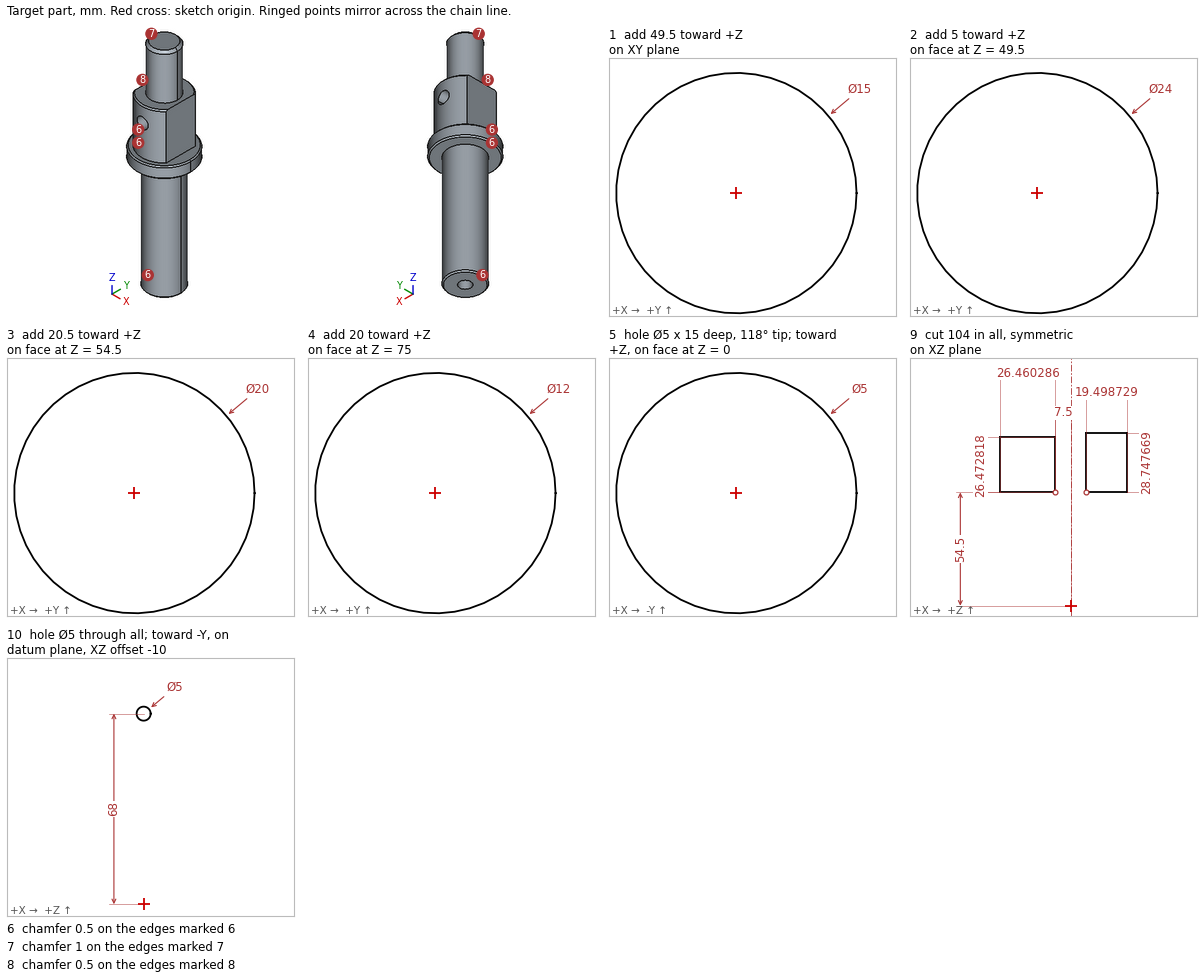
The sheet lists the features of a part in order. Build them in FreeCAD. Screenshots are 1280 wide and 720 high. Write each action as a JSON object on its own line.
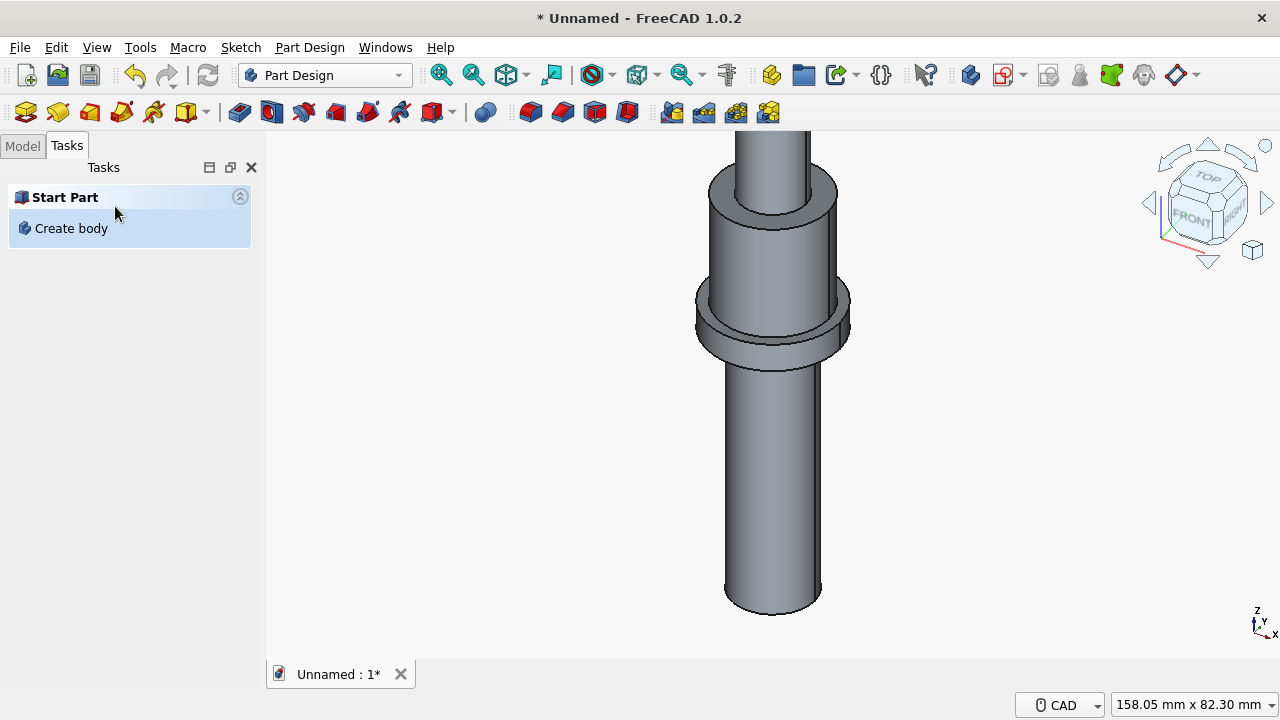
{"action": "left_click", "coordinate": [442, 76]}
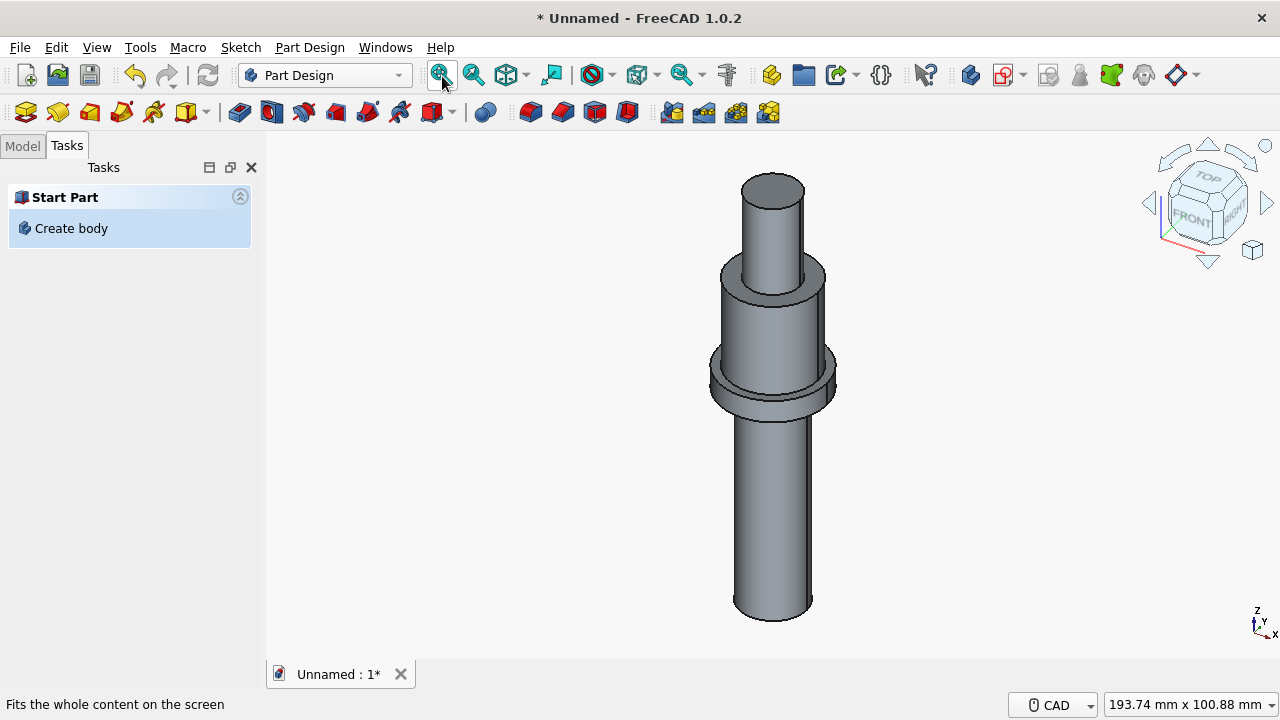
{"action": "key", "text": "5"}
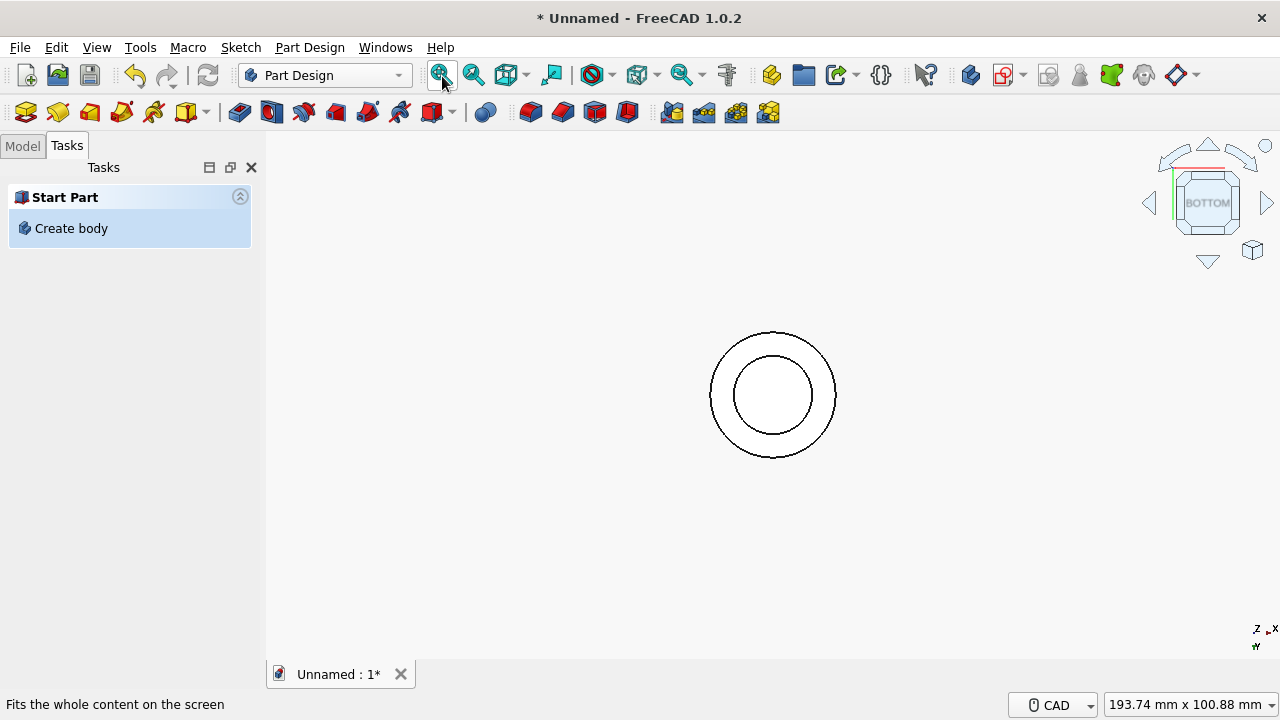
{"action": "left_click", "coordinate": [442, 76]}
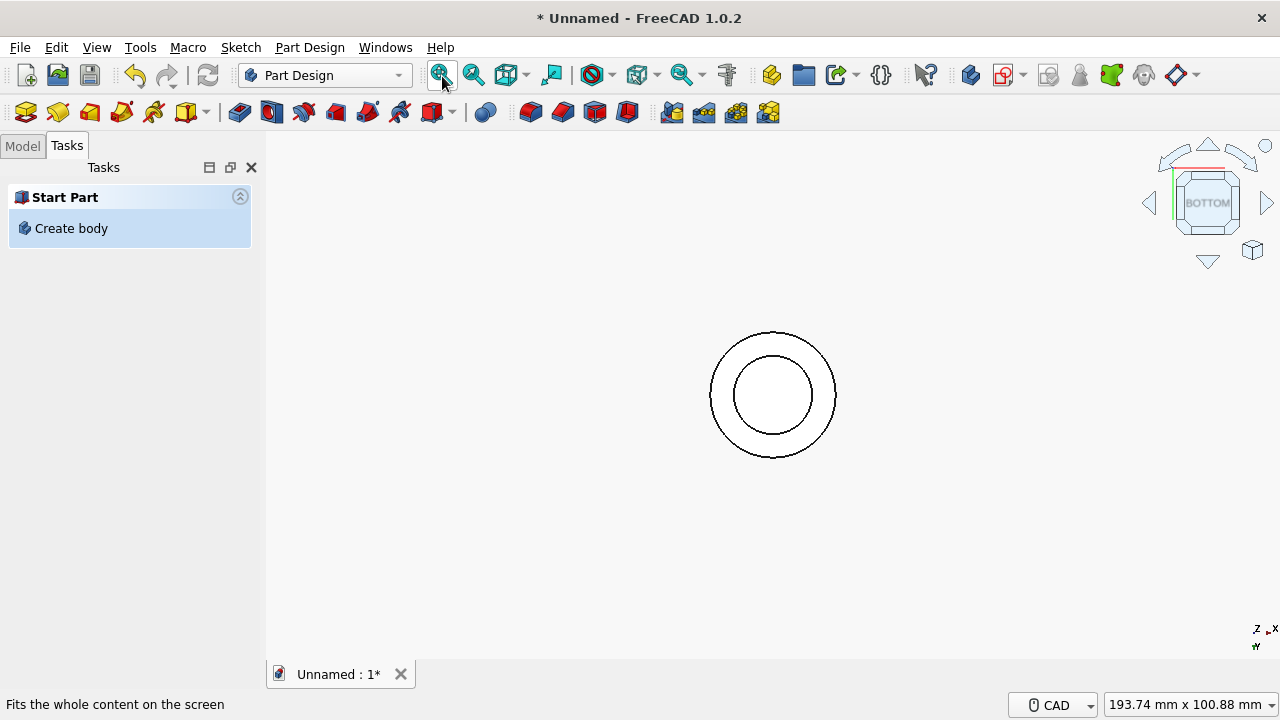
{"action": "left_click", "coordinate": [773, 394]}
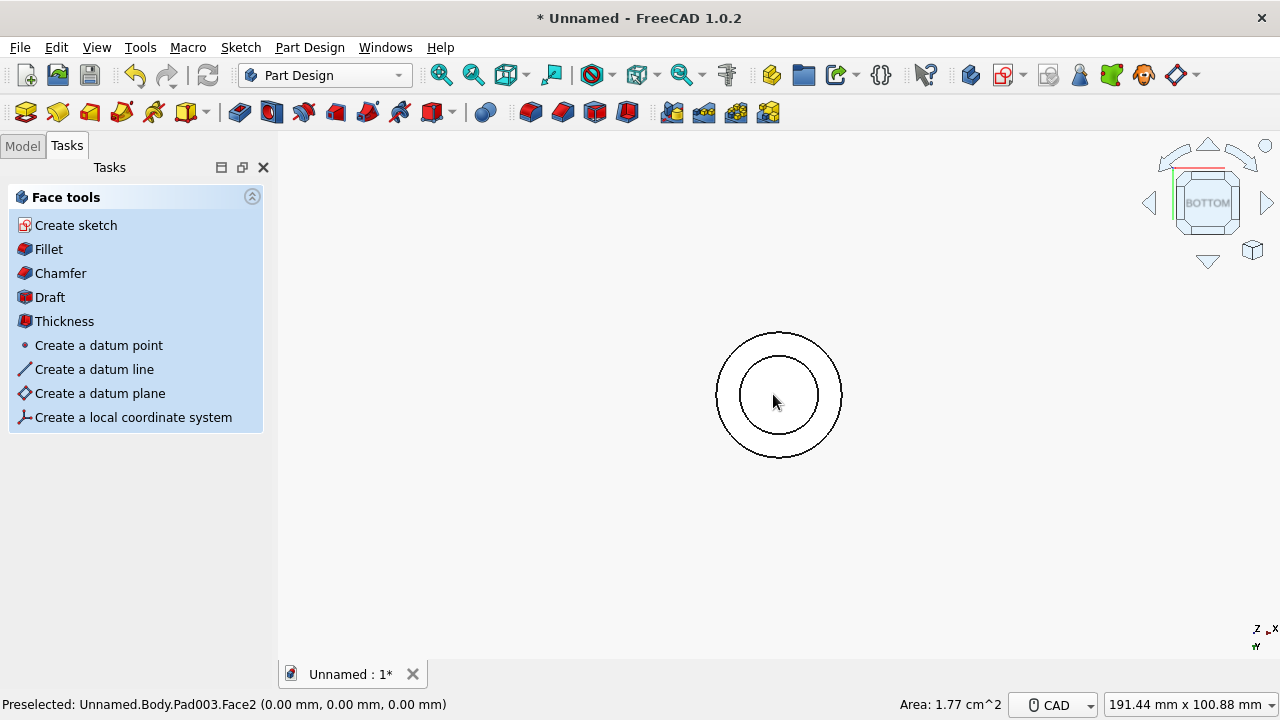
{"action": "left_click", "coordinate": [1004, 76]}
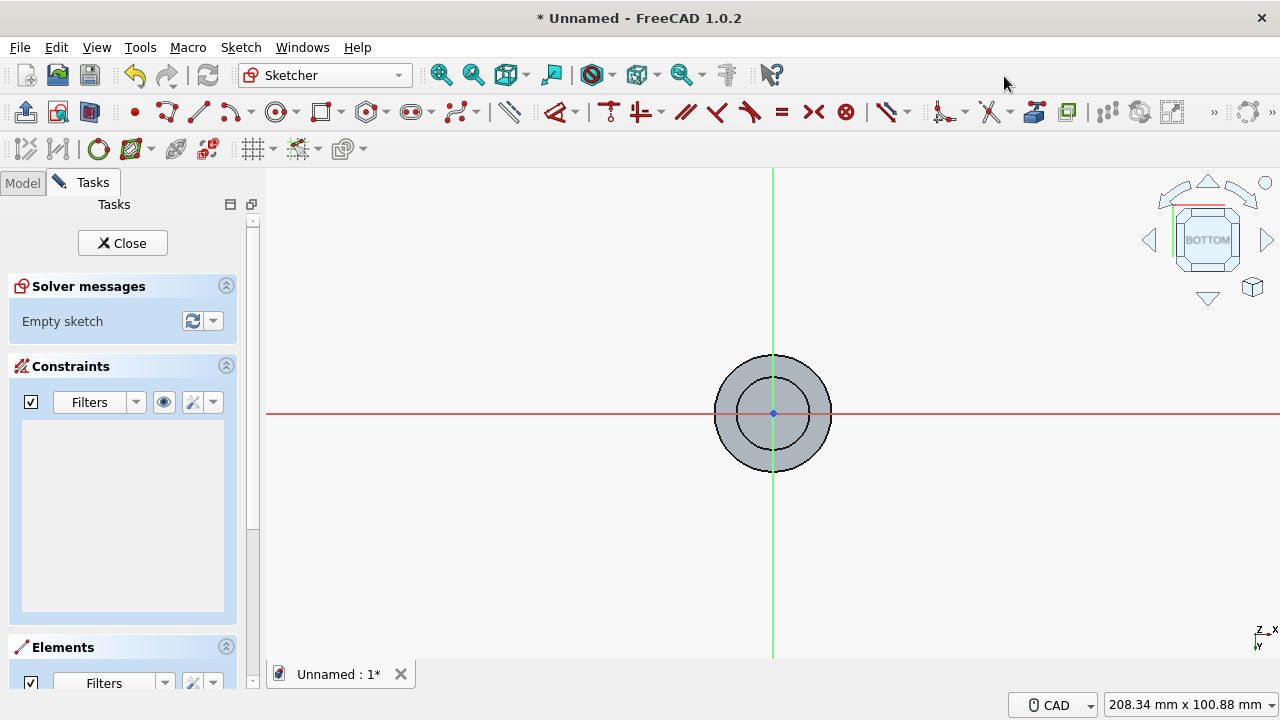
{"action": "scroll", "coordinate": [778, 414], "scroll_direction": "up", "scroll_amount": 13}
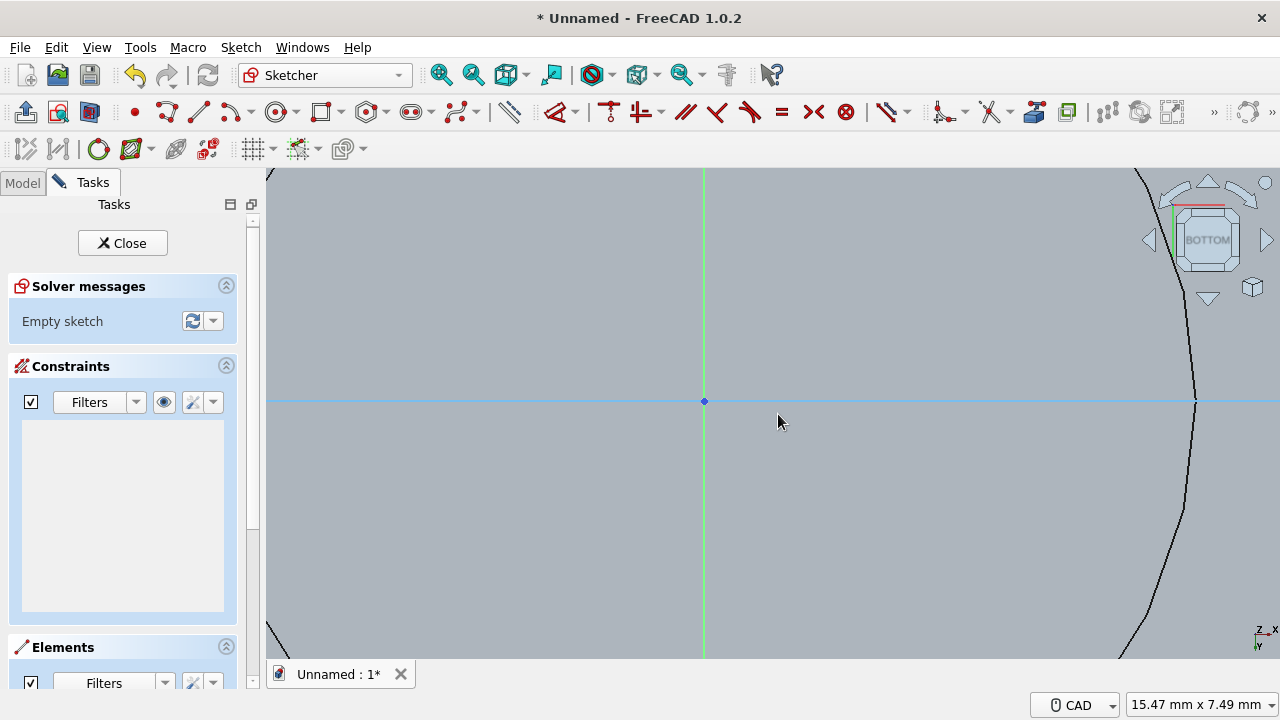
{"action": "left_click", "coordinate": [276, 112]}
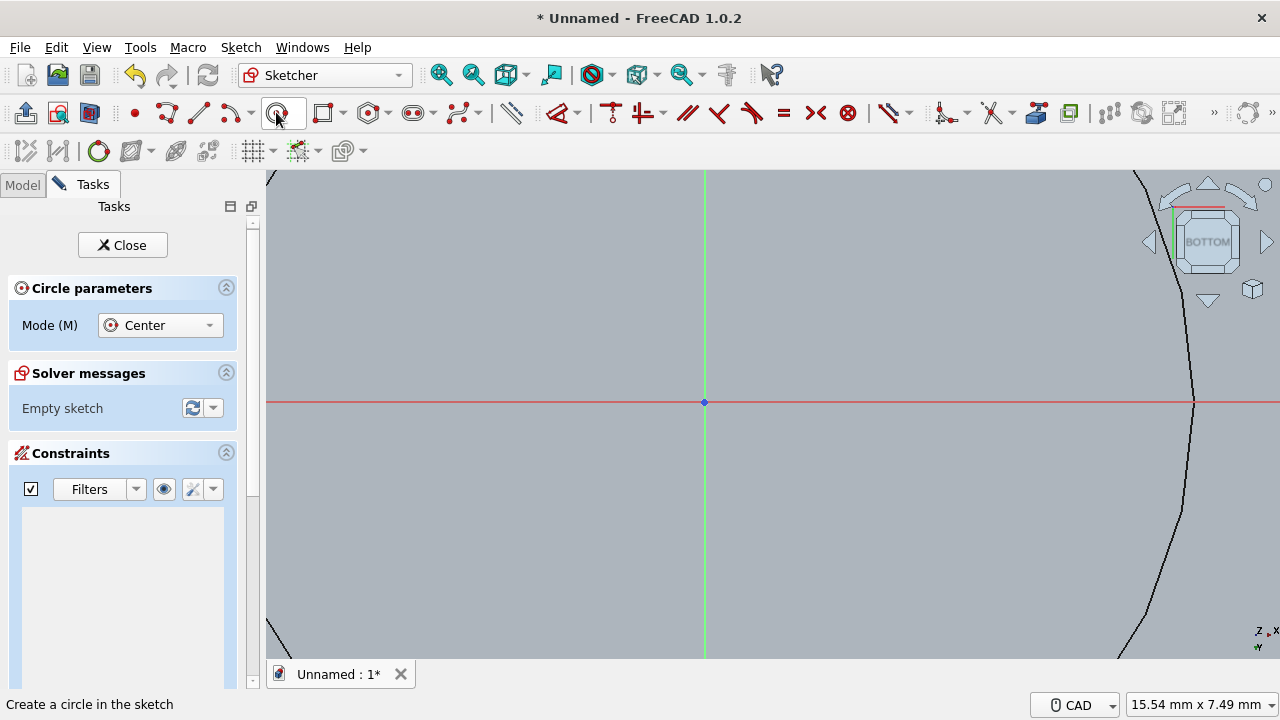
{"action": "left_click", "coordinate": [705, 402]}
{"action": "mouse_move", "coordinate": [820, 287]}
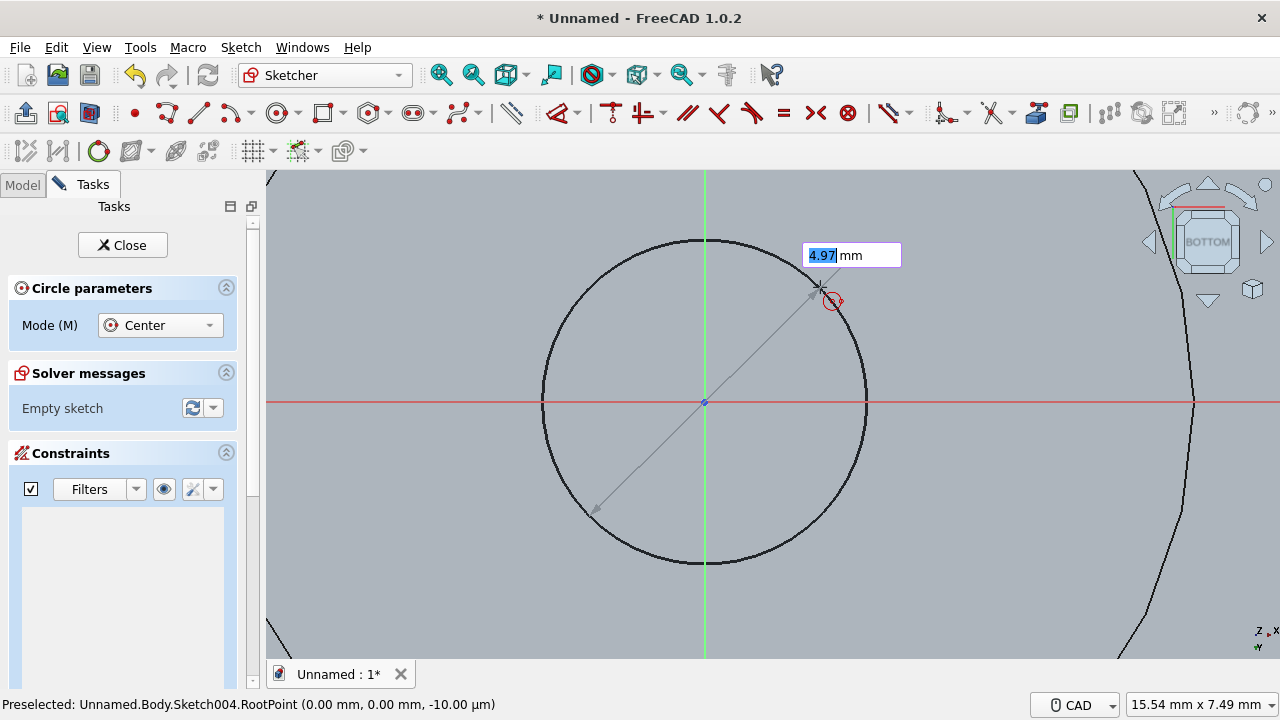
{"action": "type", "text": "5"}
{"action": "key", "text": "Return"}
{"action": "key", "text": "Escape"}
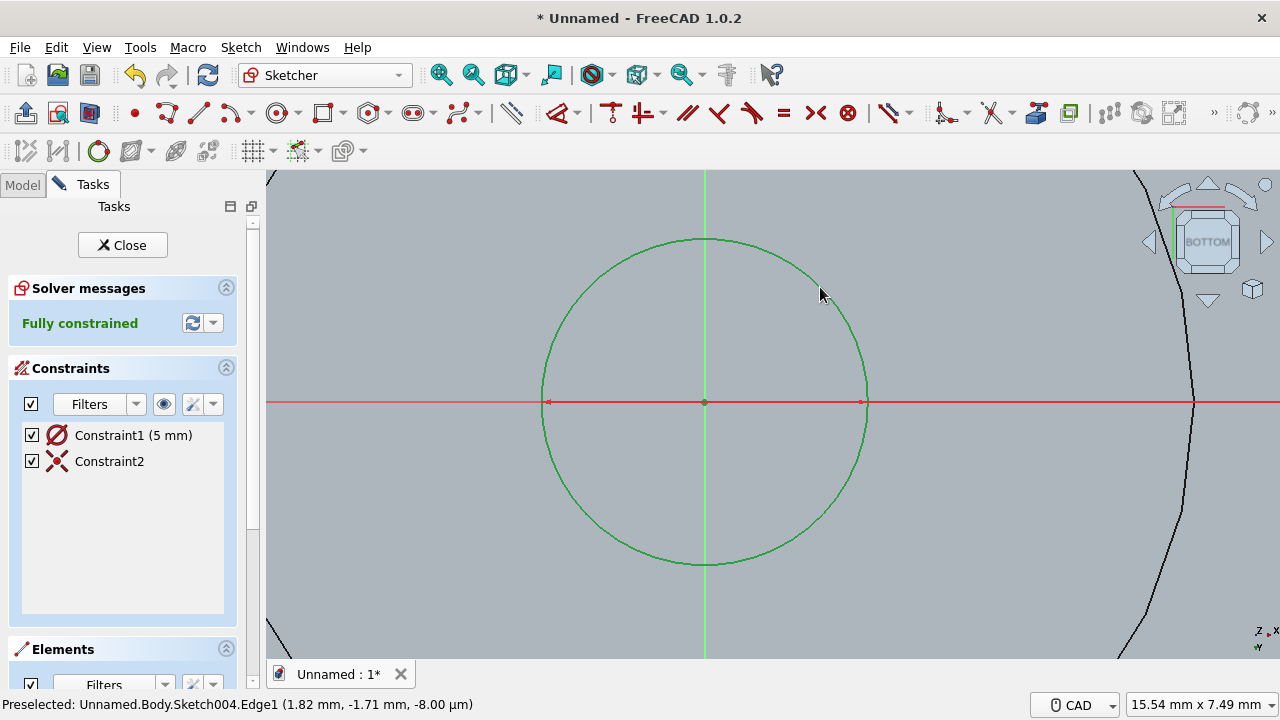
{"action": "left_click", "coordinate": [123, 245]}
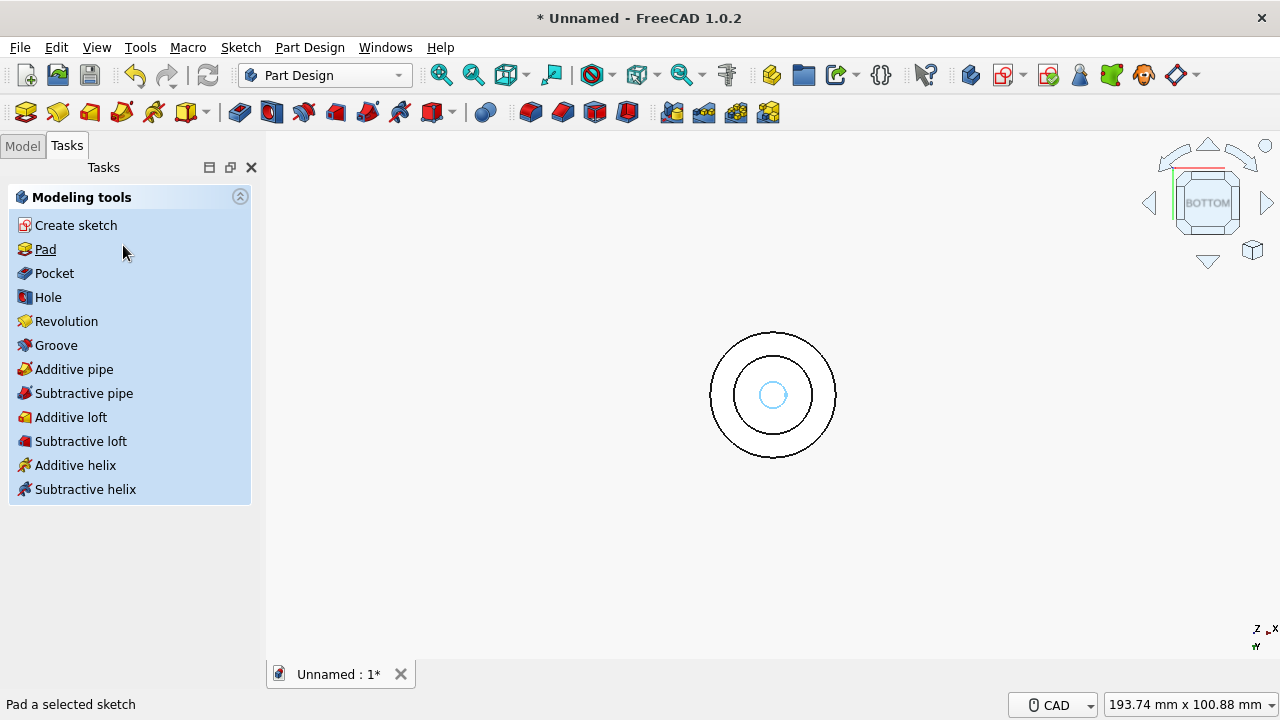
{"action": "left_click", "coordinate": [272, 112]}